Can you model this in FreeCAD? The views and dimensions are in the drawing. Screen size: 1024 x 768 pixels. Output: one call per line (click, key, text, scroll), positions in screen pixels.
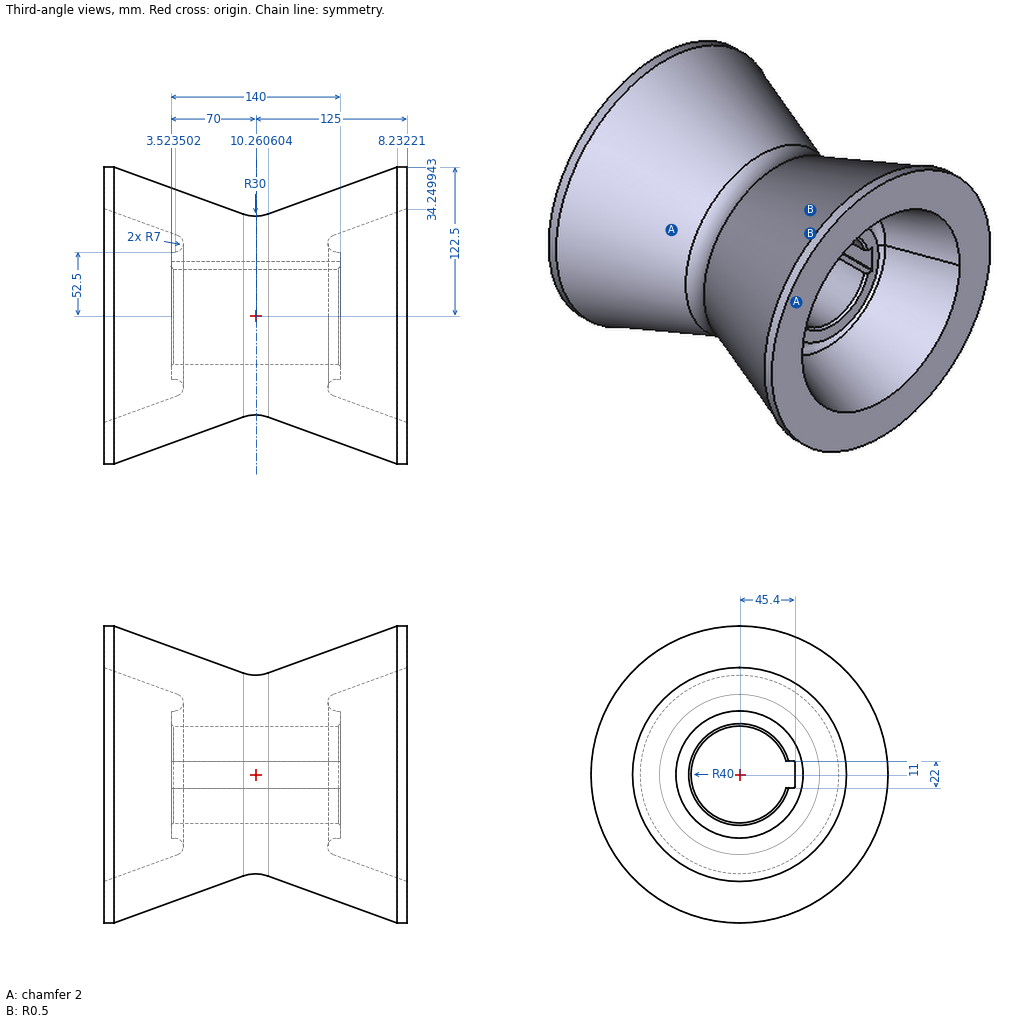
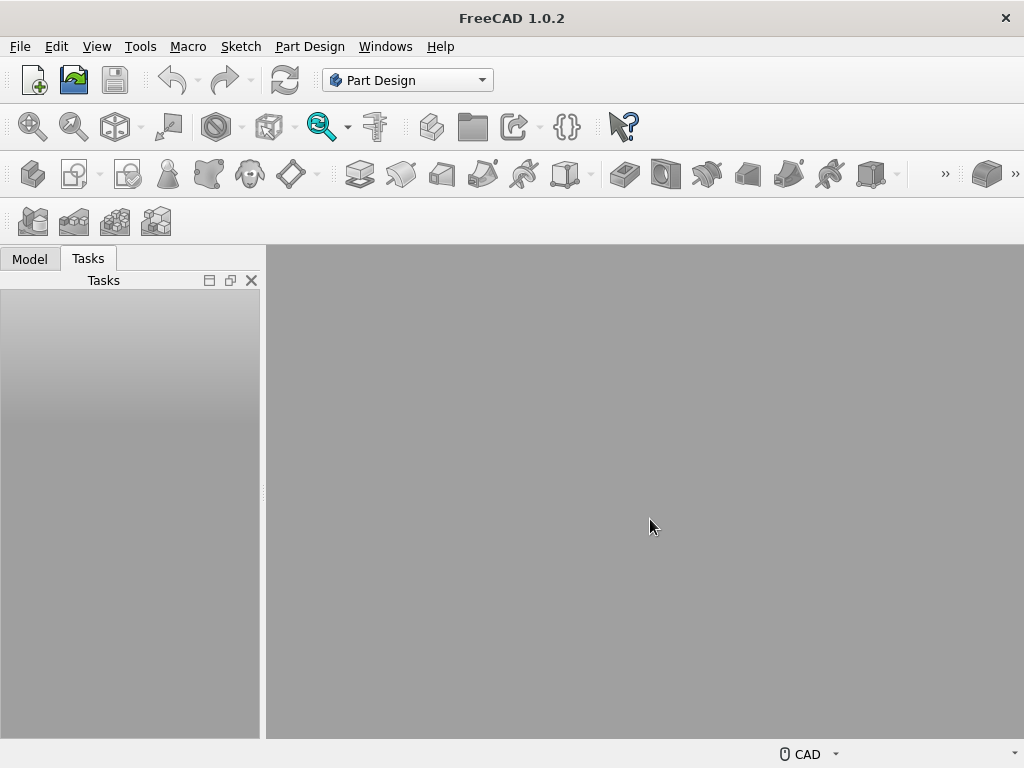
click(33, 80)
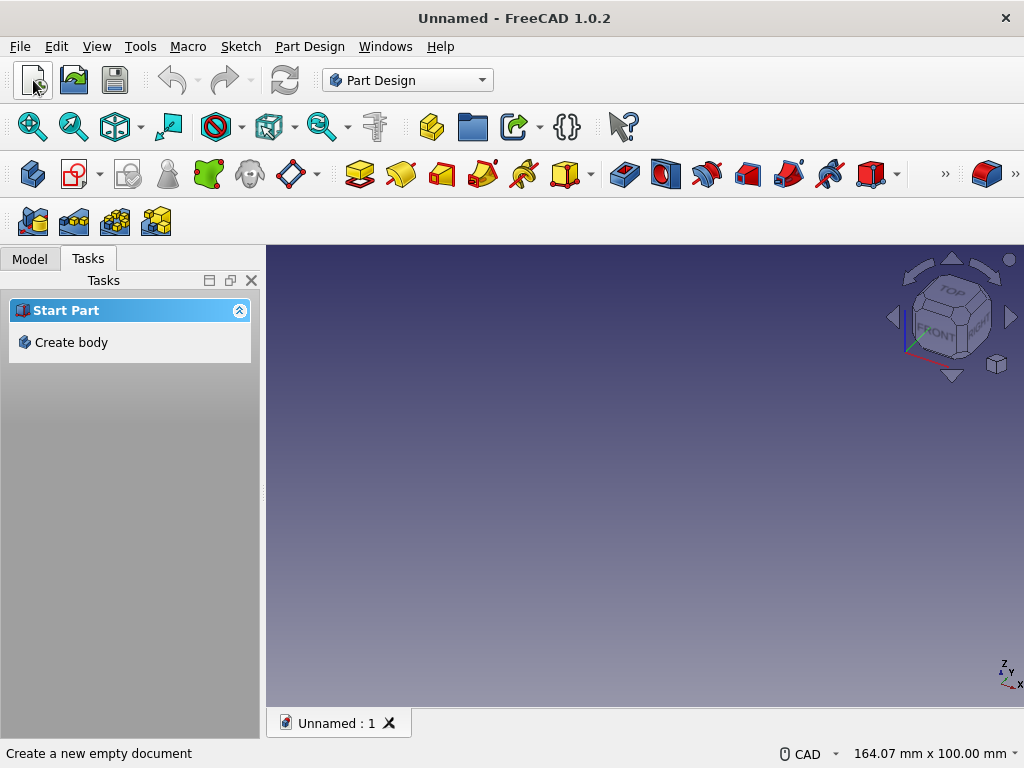
click(74, 174)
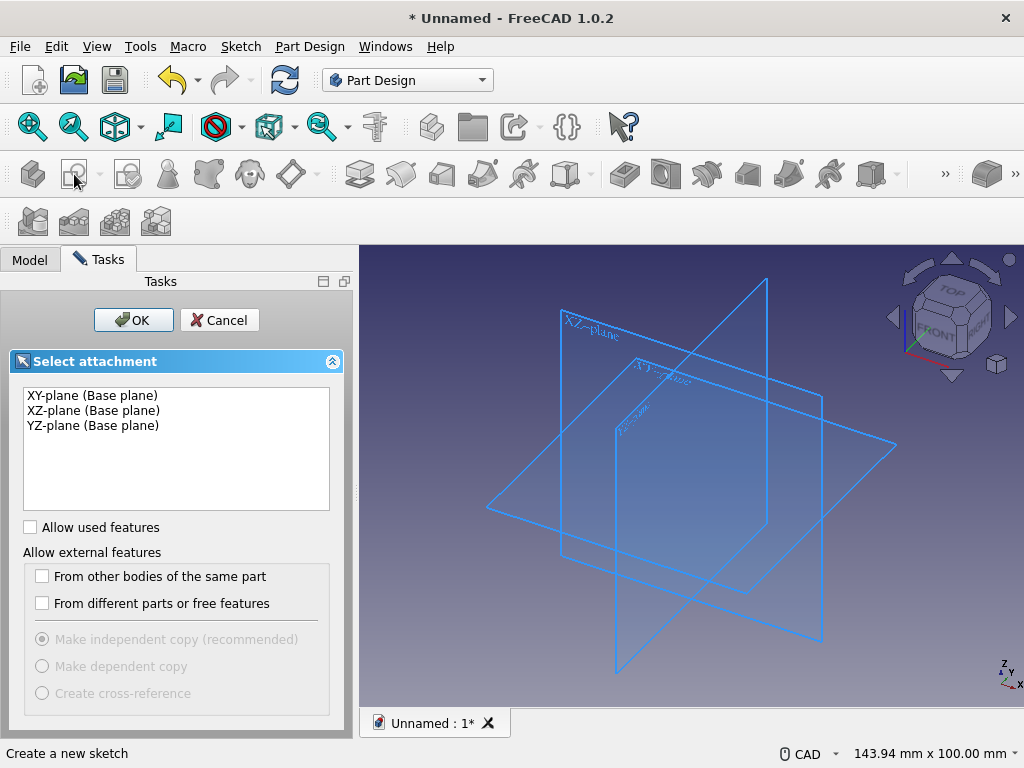
click(84, 396)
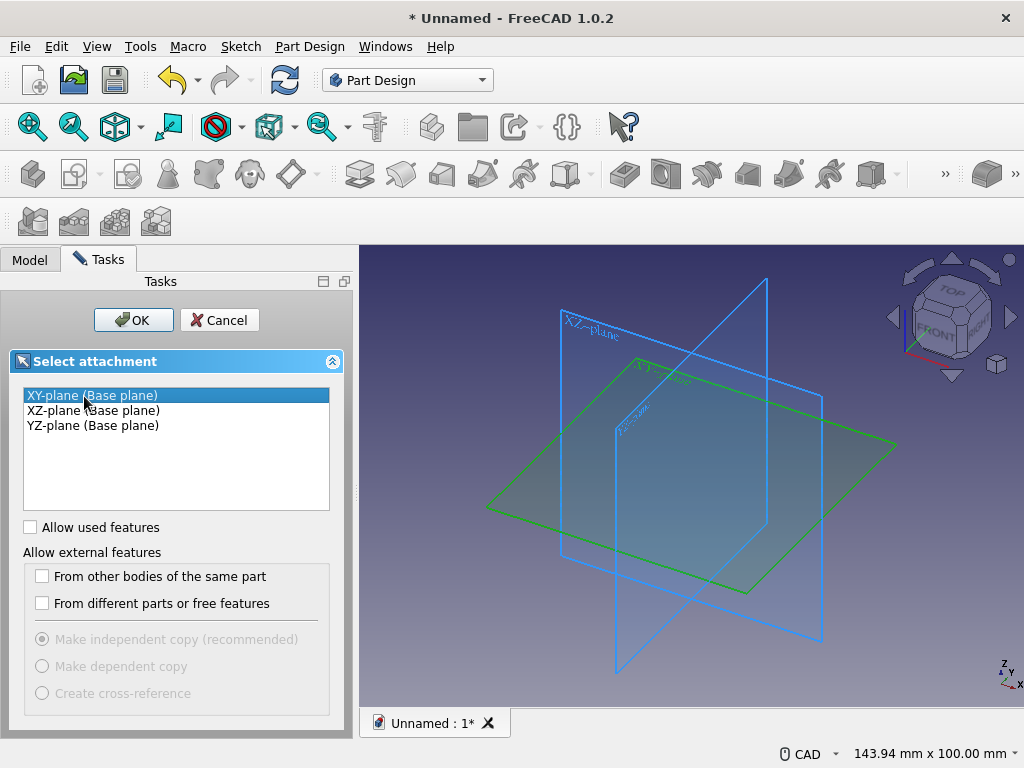
click(134, 320)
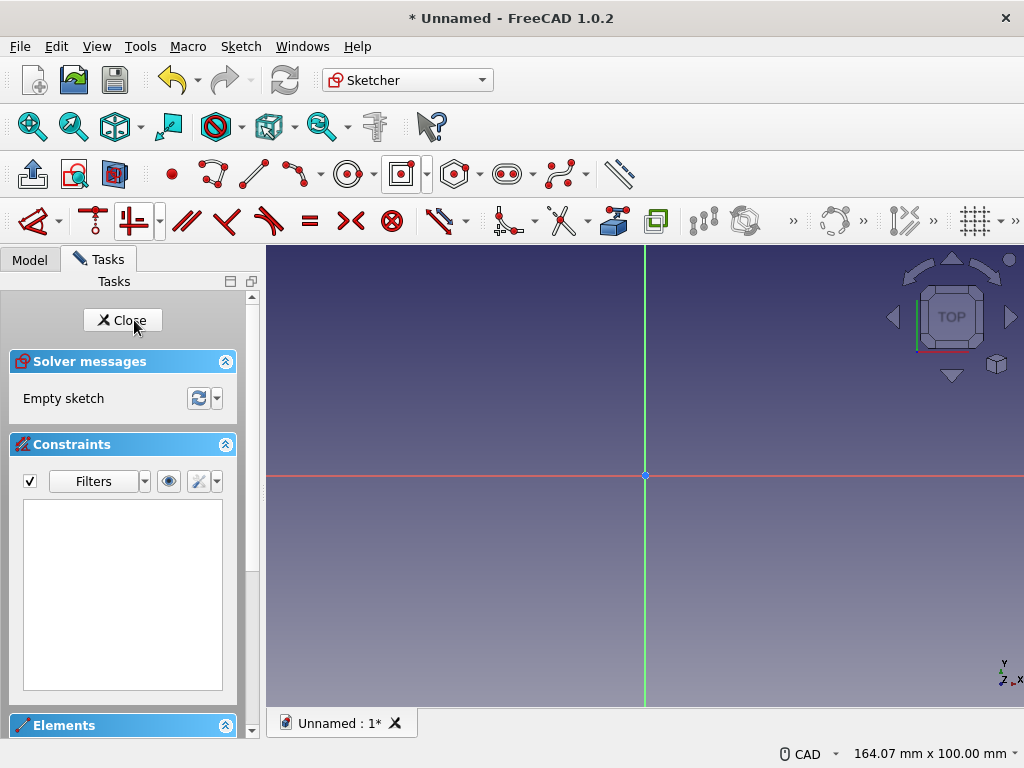
scroll(537, 641, down, 5)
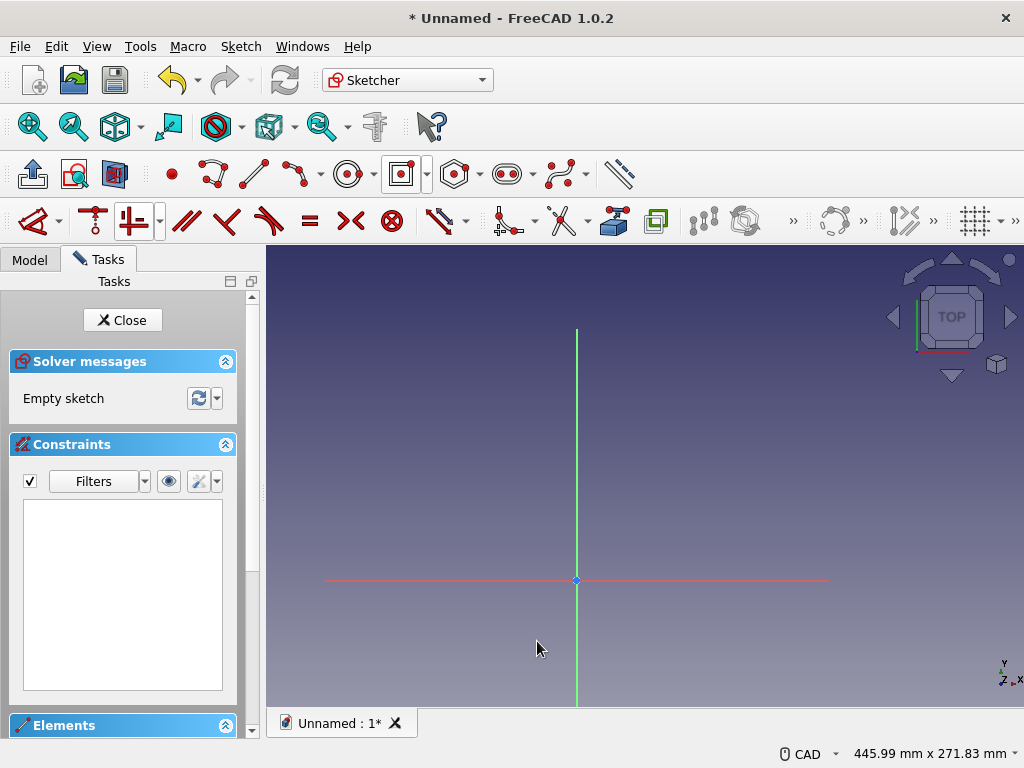
click(213, 174)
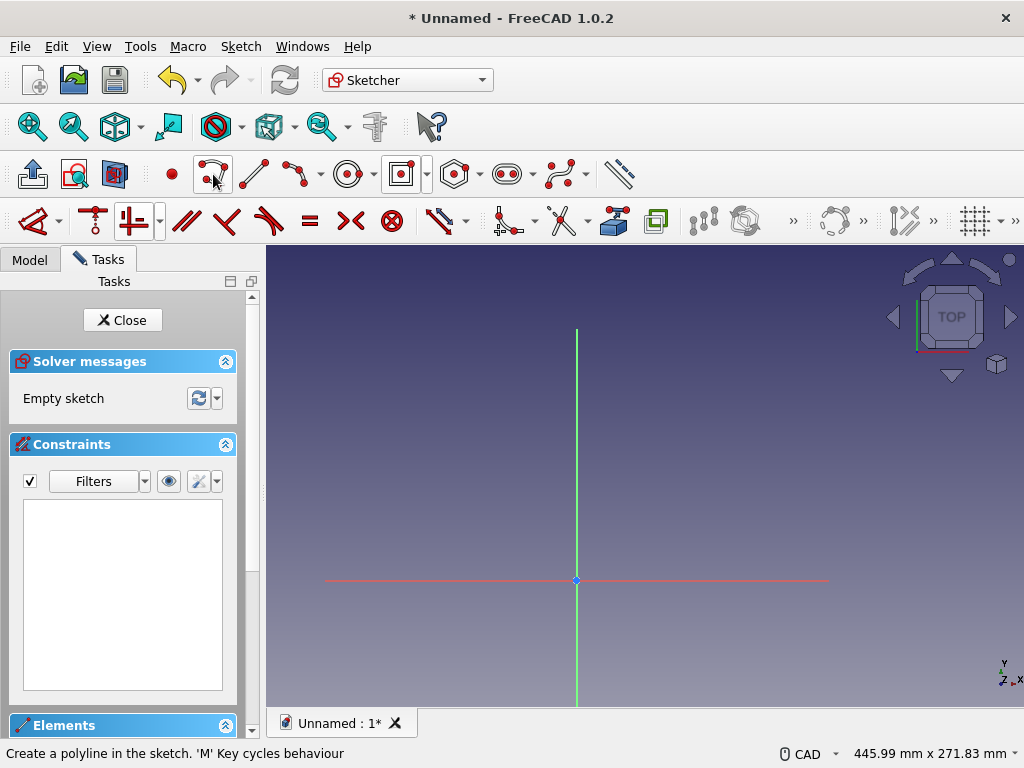
click(464, 492)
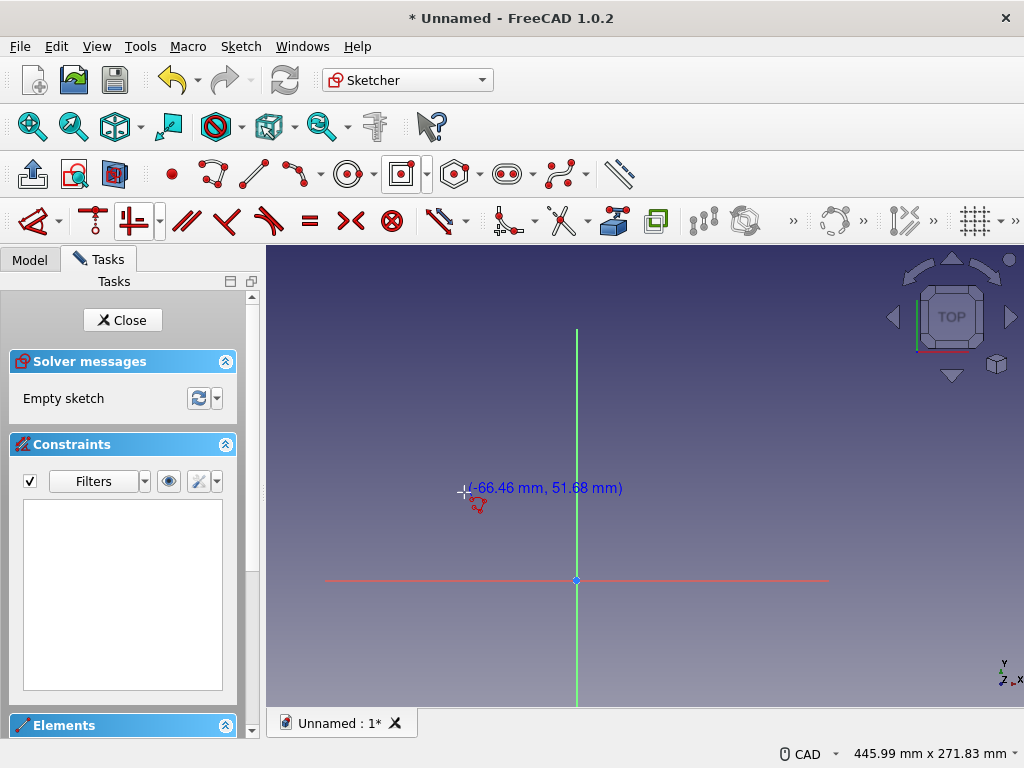
scroll(458, 492, up, 5)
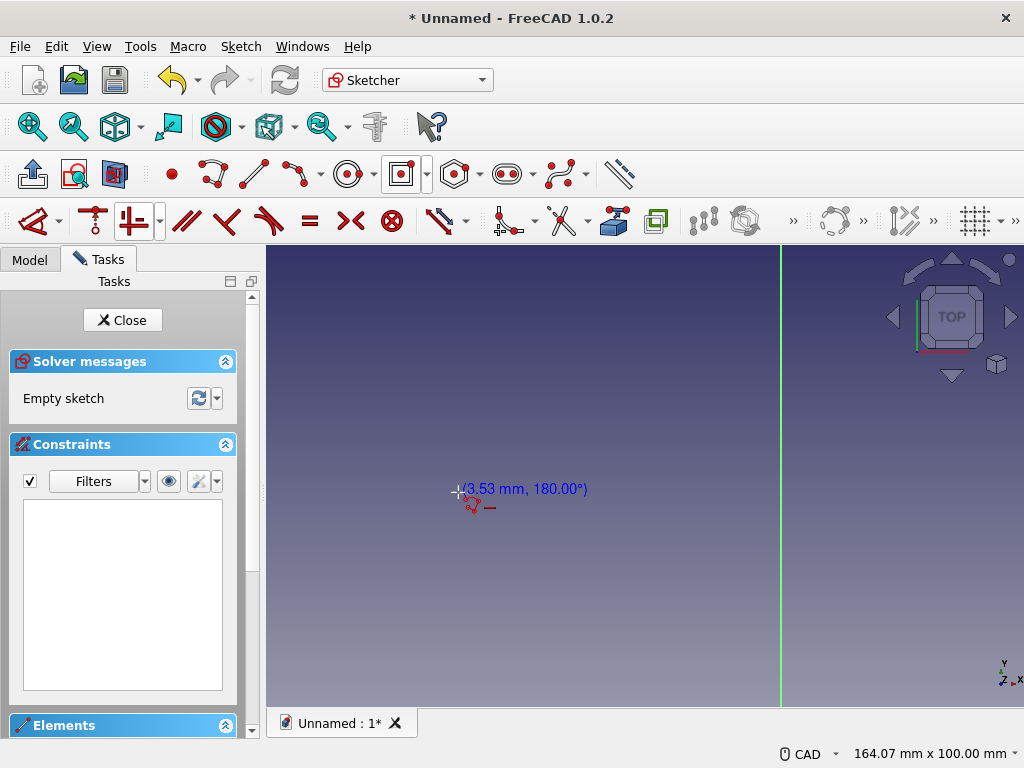
click(458, 491)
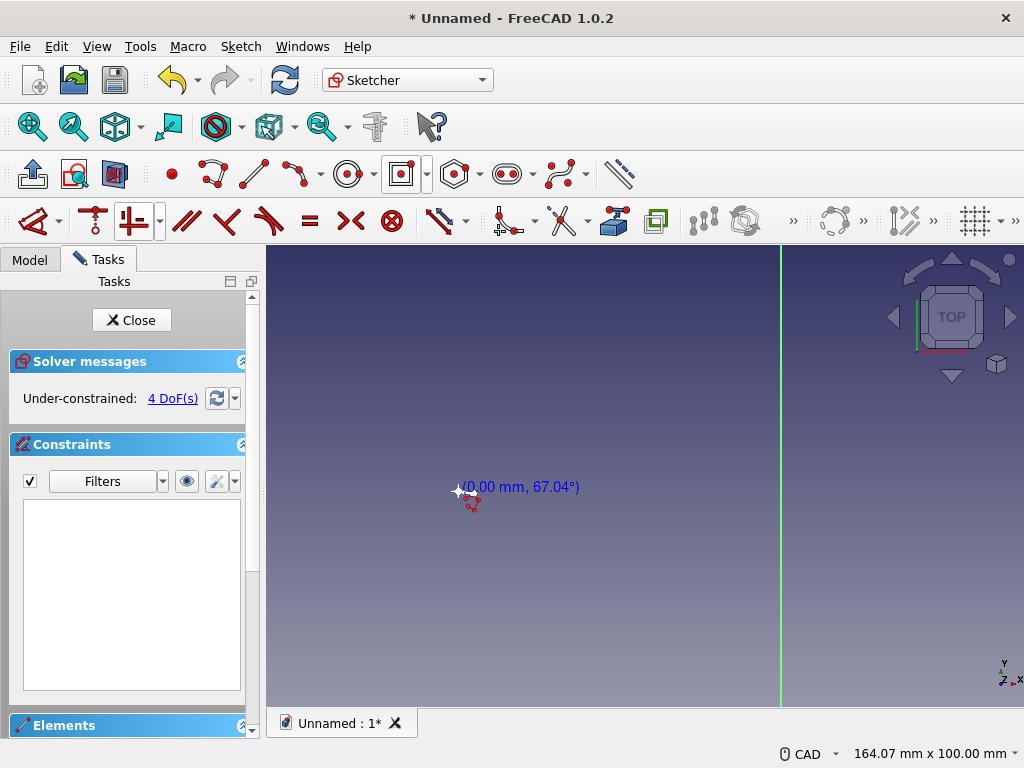
scroll(458, 491, down, 5)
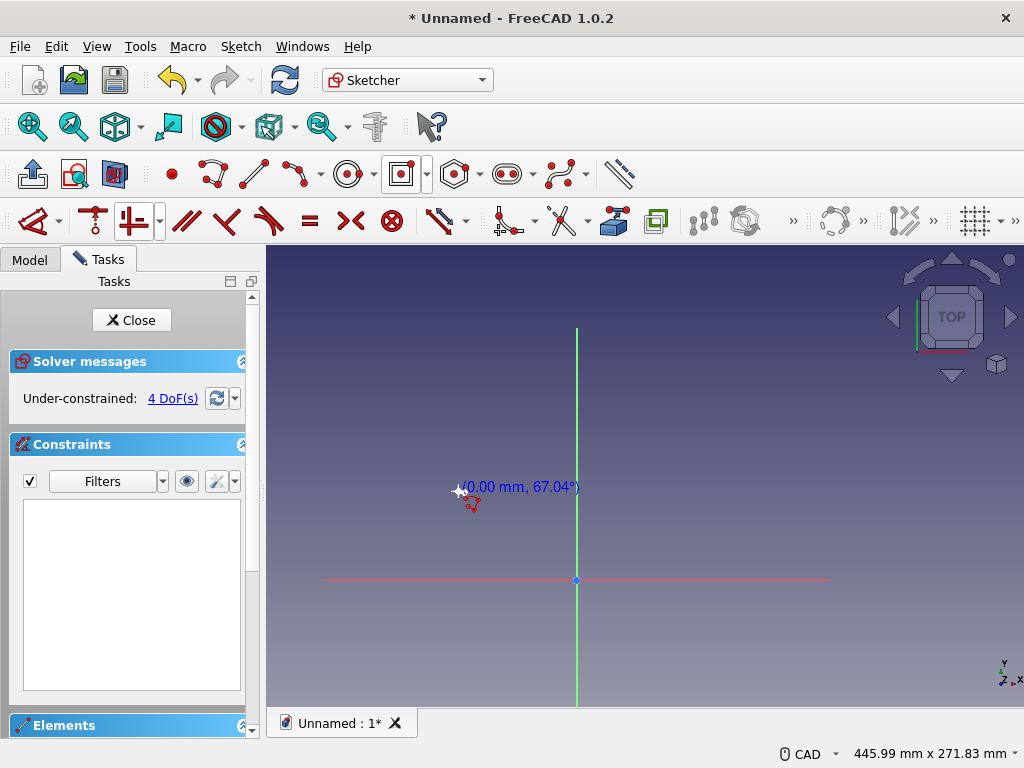
click(458, 580)
click(696, 571)
click(696, 491)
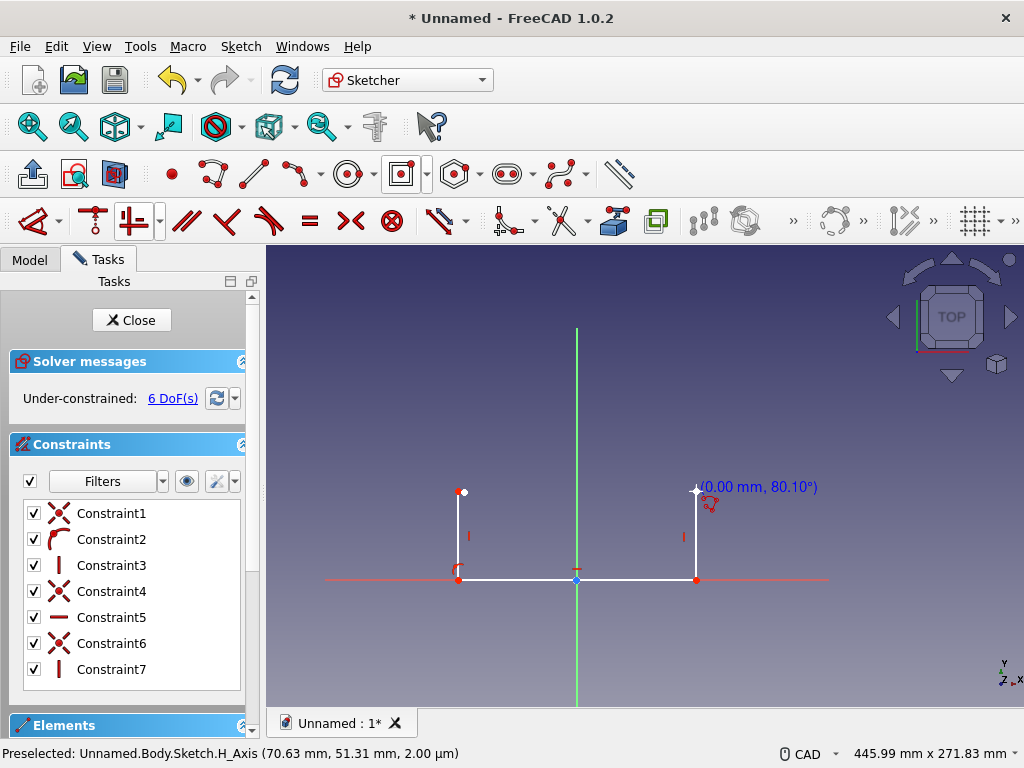
scroll(690, 491, up, 5)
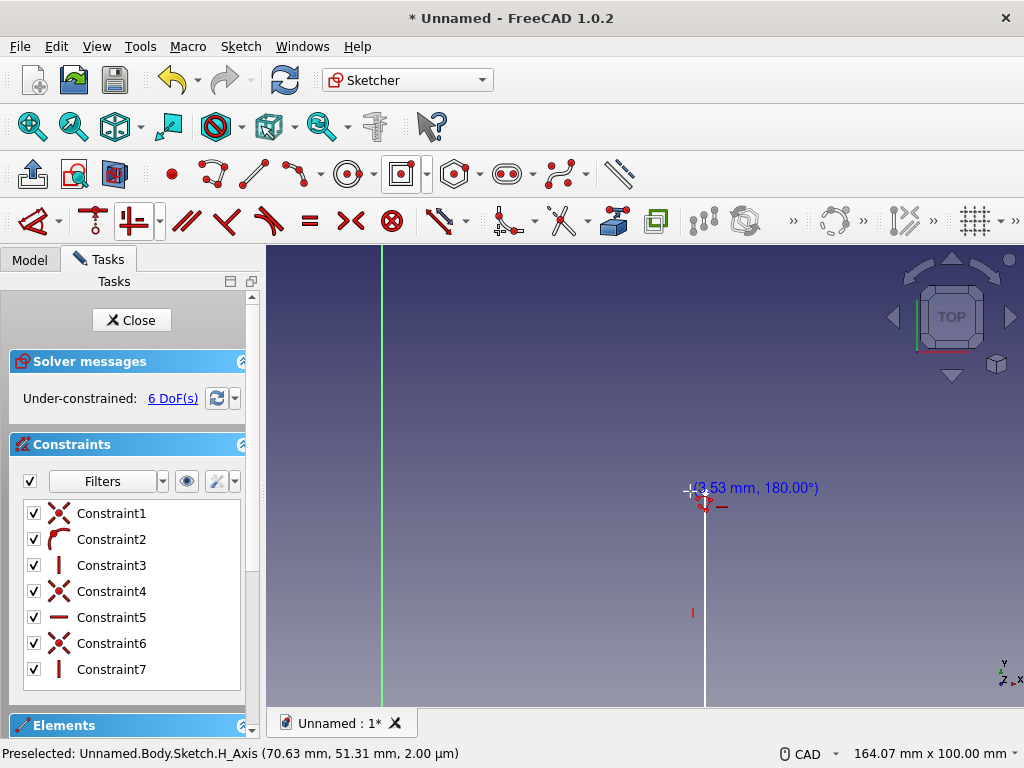
click(689, 490)
right_click(689, 490)